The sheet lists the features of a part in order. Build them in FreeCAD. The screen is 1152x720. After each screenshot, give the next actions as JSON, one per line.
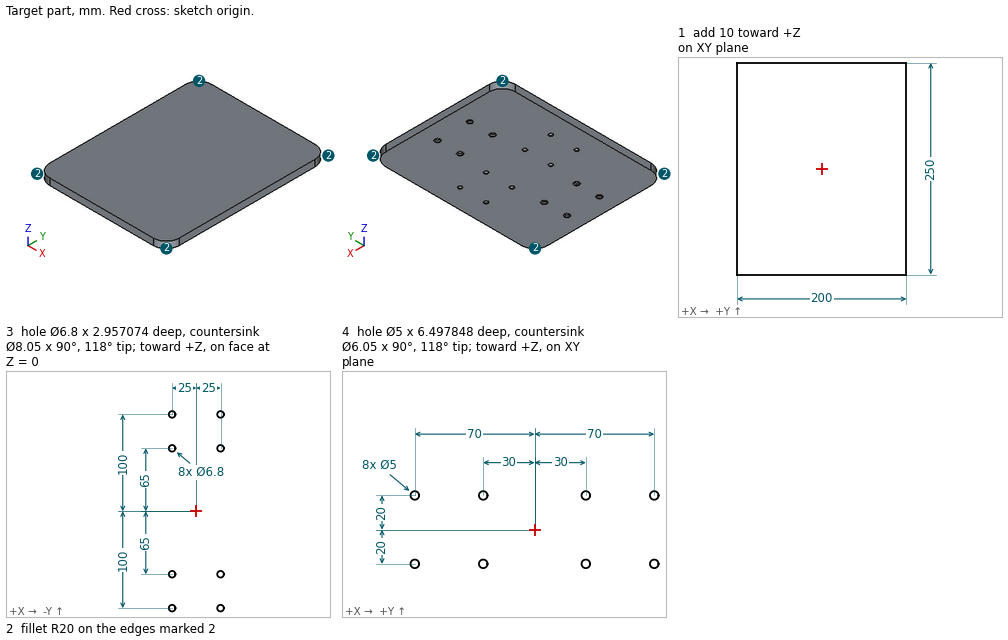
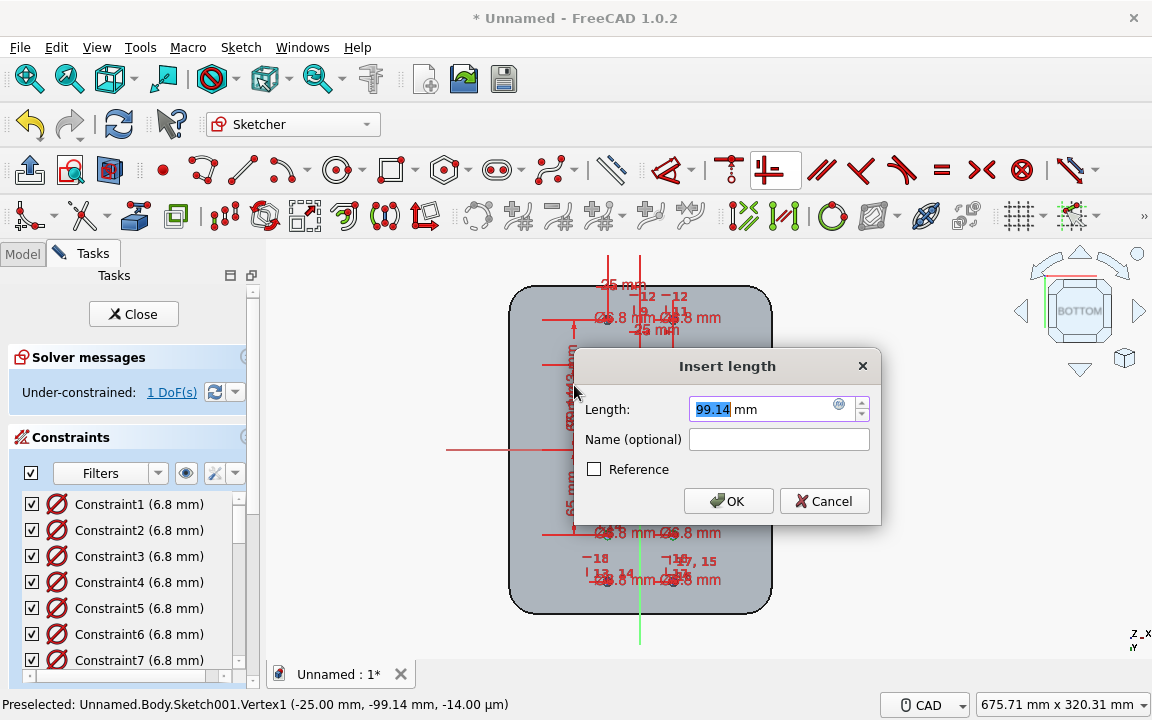
{"action": "type", "text": "100"}
{"action": "key", "text": "Return"}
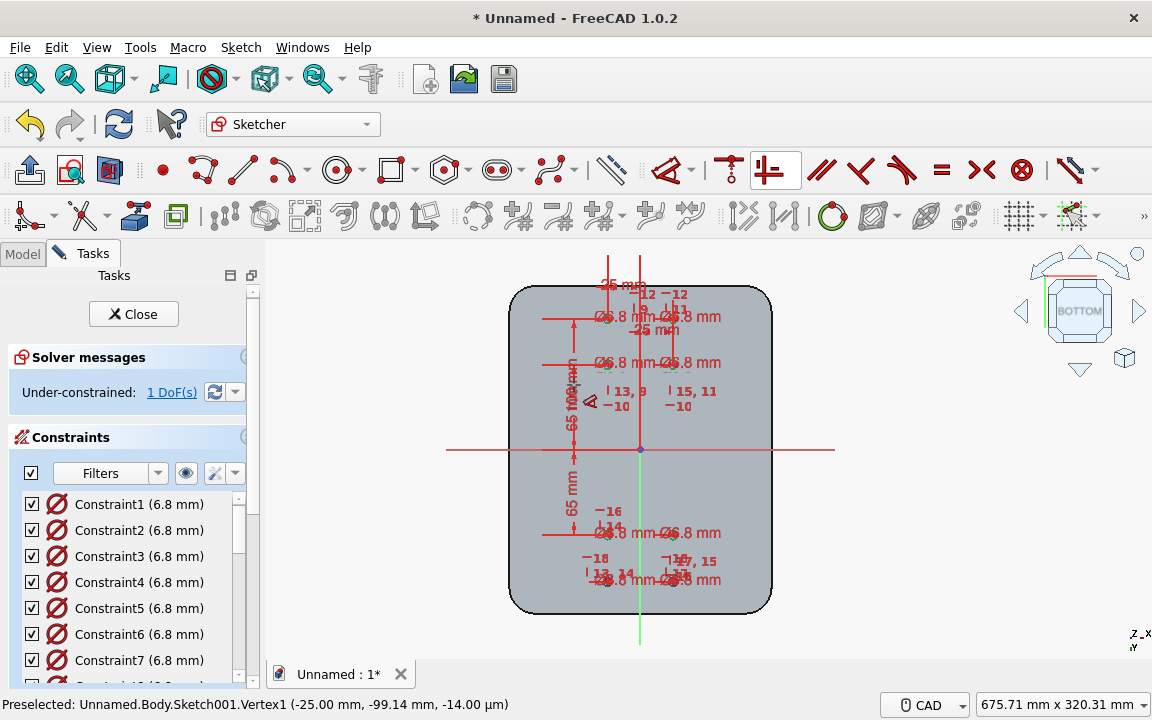
{"action": "left_click", "coordinate": [608, 582]}
{"action": "left_click", "coordinate": [574, 516]}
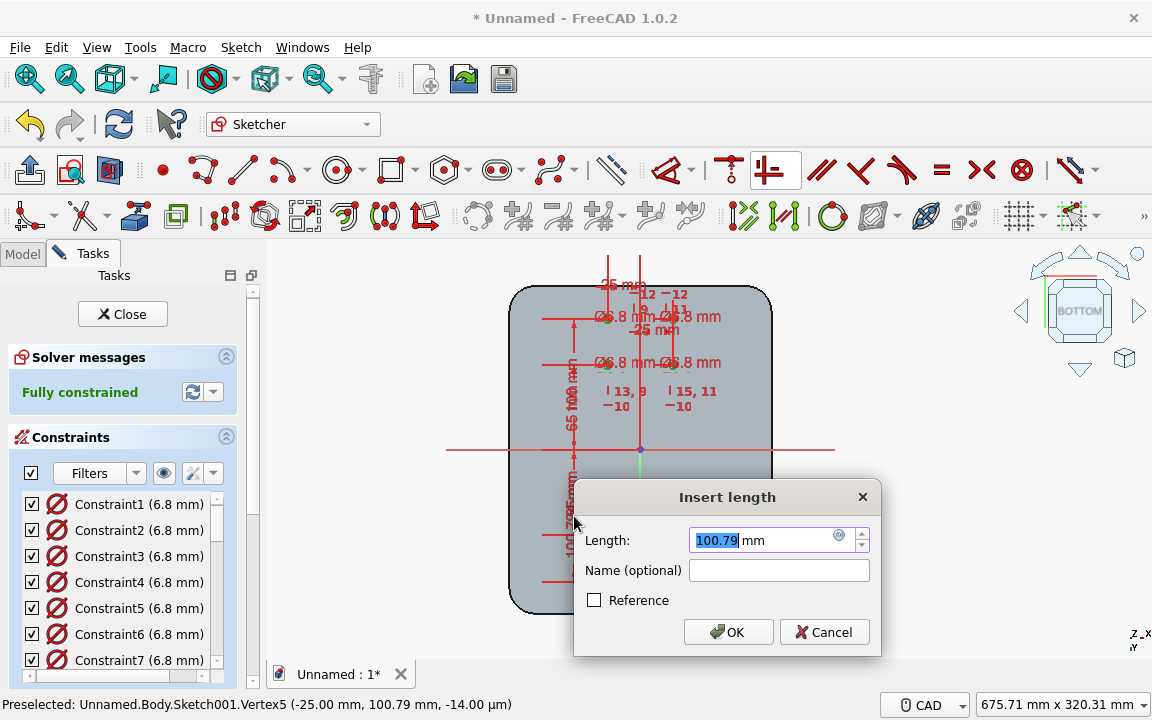
{"action": "type", "text": "100"}
{"action": "key", "text": "Return"}
{"action": "key", "text": "Escape"}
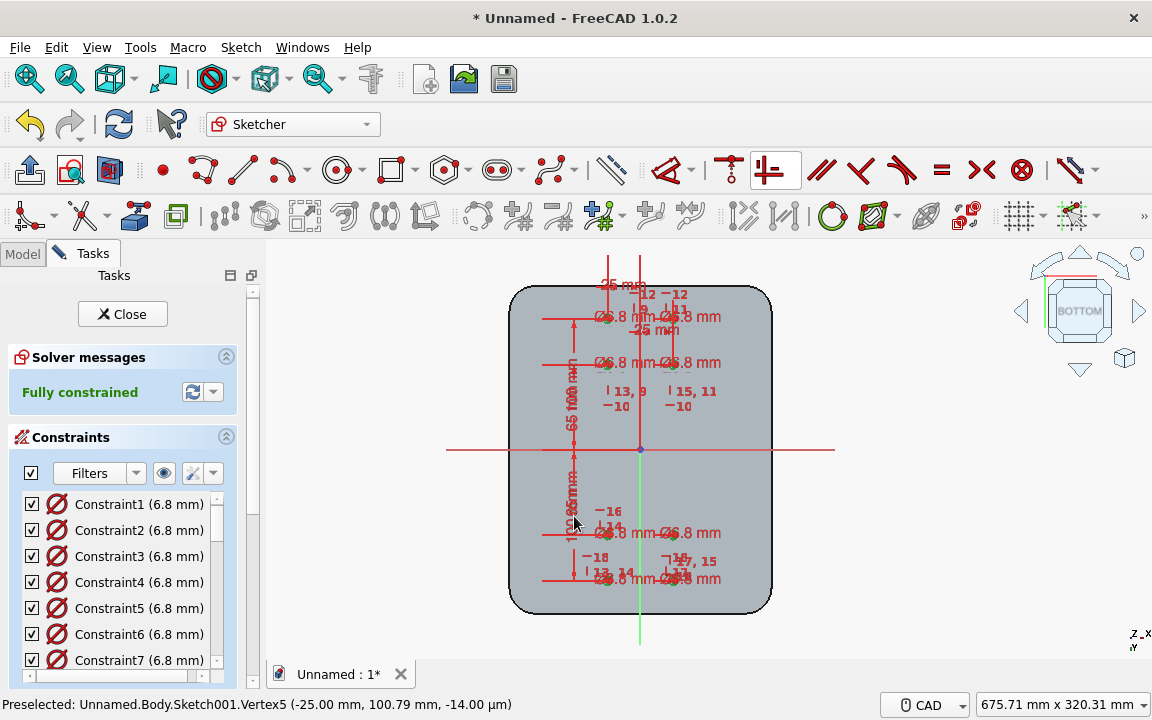
{"action": "left_click", "coordinate": [123, 314]}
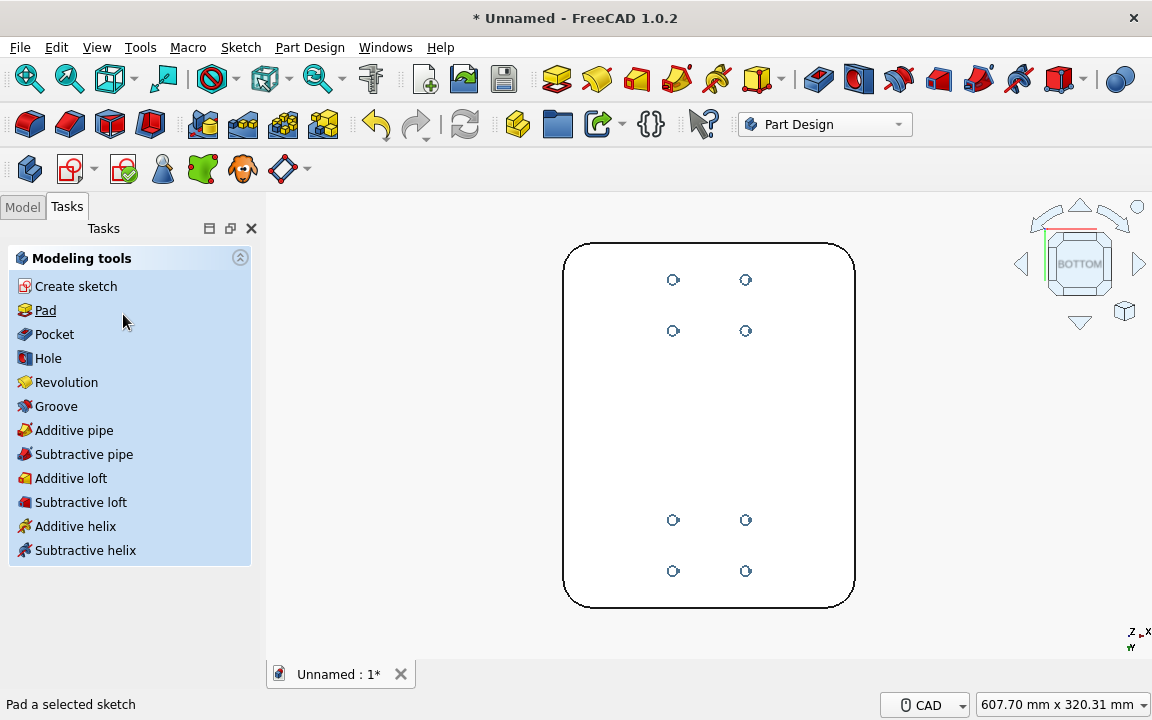
{"action": "left_click", "coordinate": [860, 80]}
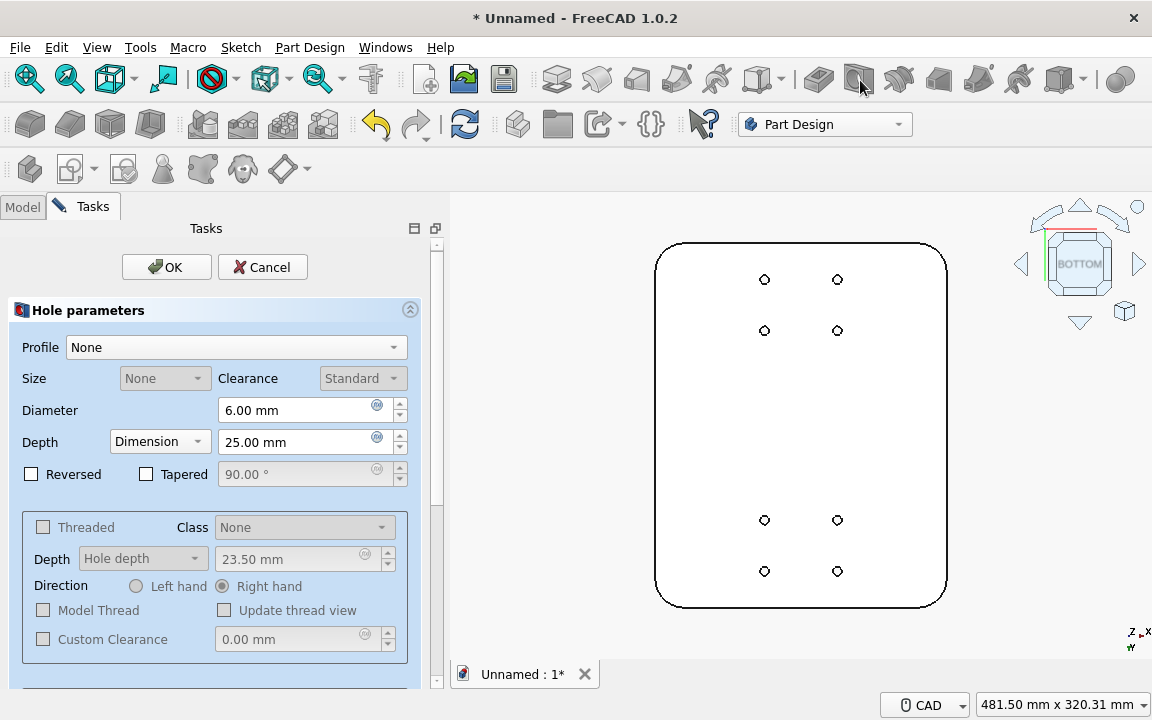
{"action": "triple_click", "coordinate": [305, 410]}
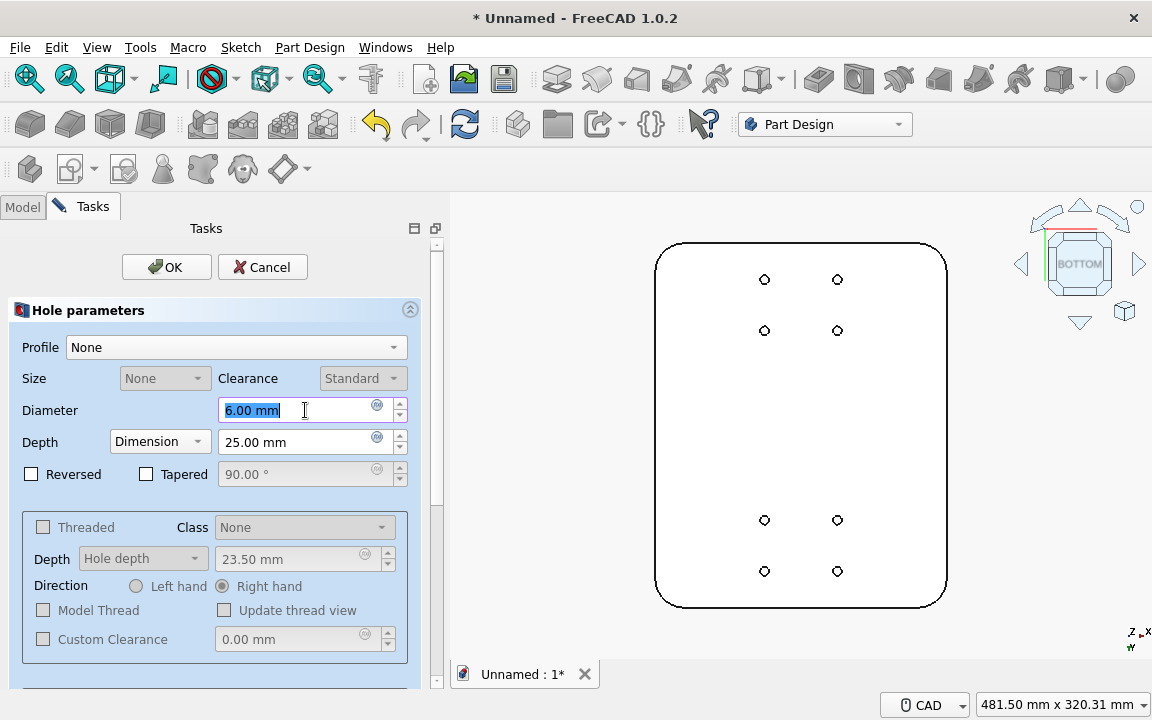
{"action": "type", "text": "6.8"}
{"action": "key", "text": "Tab"}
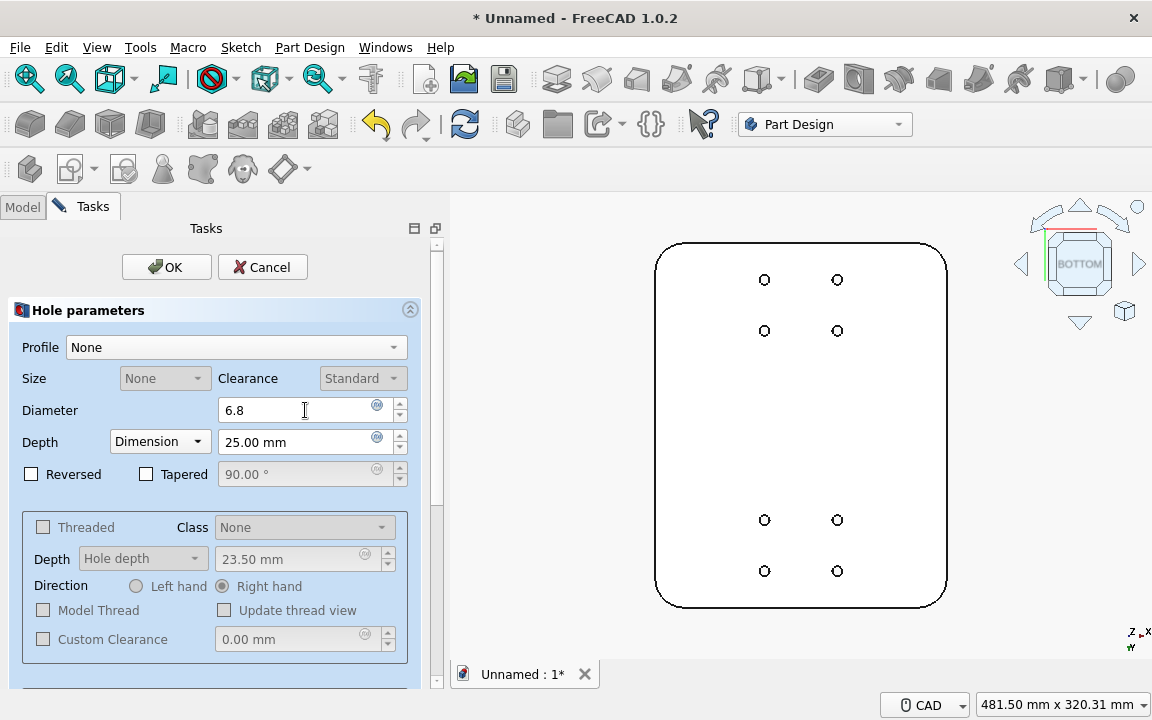
{"action": "triple_click", "coordinate": [305, 442]}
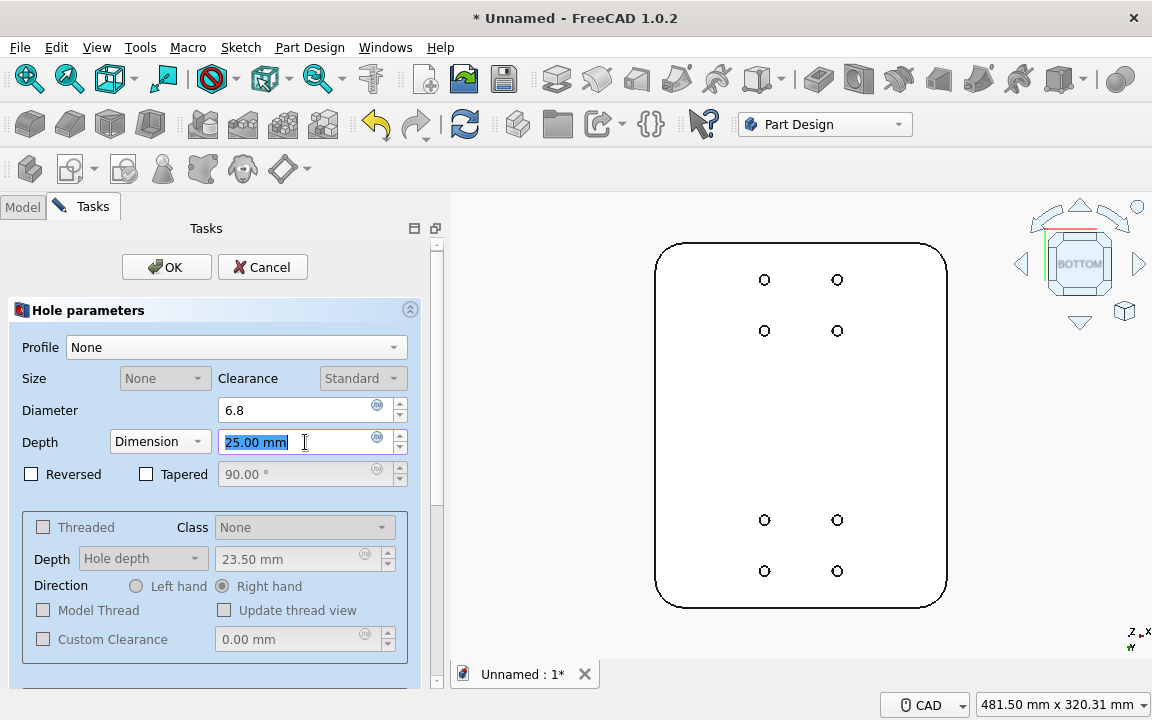
{"action": "type", "text": "2.957074"}
{"action": "key", "text": "Tab"}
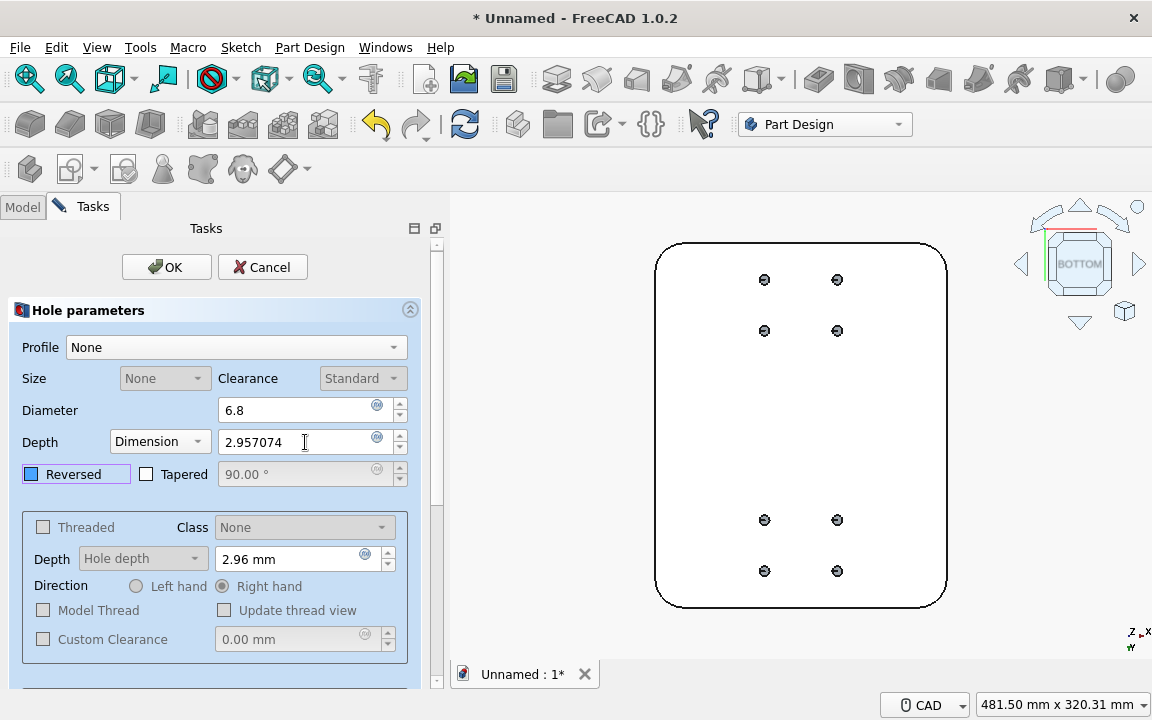
{"action": "scroll", "coordinate": [437, 463], "scroll_direction": "down", "scroll_amount": 2}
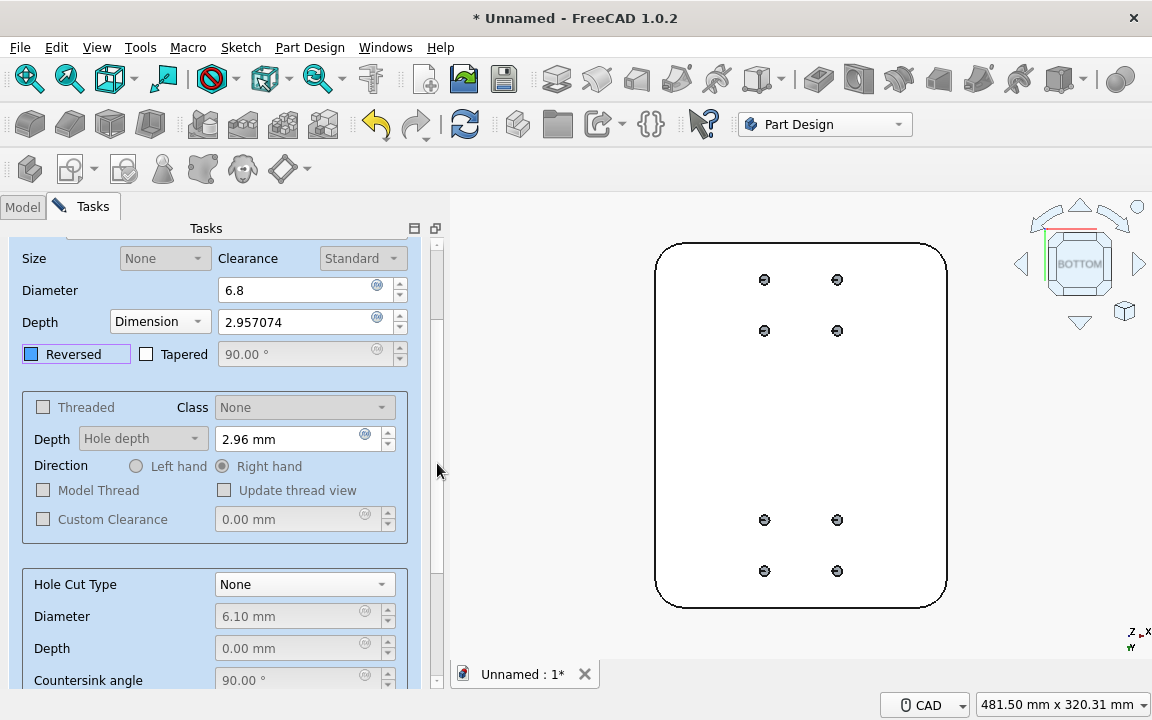
{"action": "left_click", "coordinate": [306, 584]}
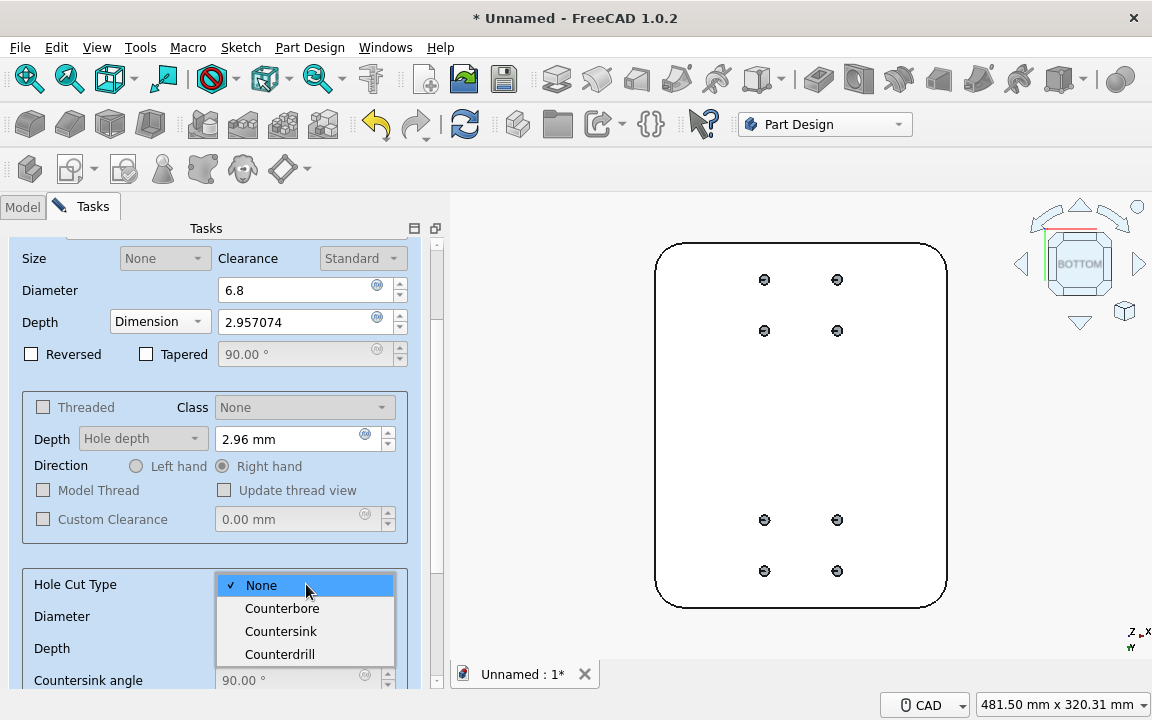
{"action": "left_click", "coordinate": [304, 632]}